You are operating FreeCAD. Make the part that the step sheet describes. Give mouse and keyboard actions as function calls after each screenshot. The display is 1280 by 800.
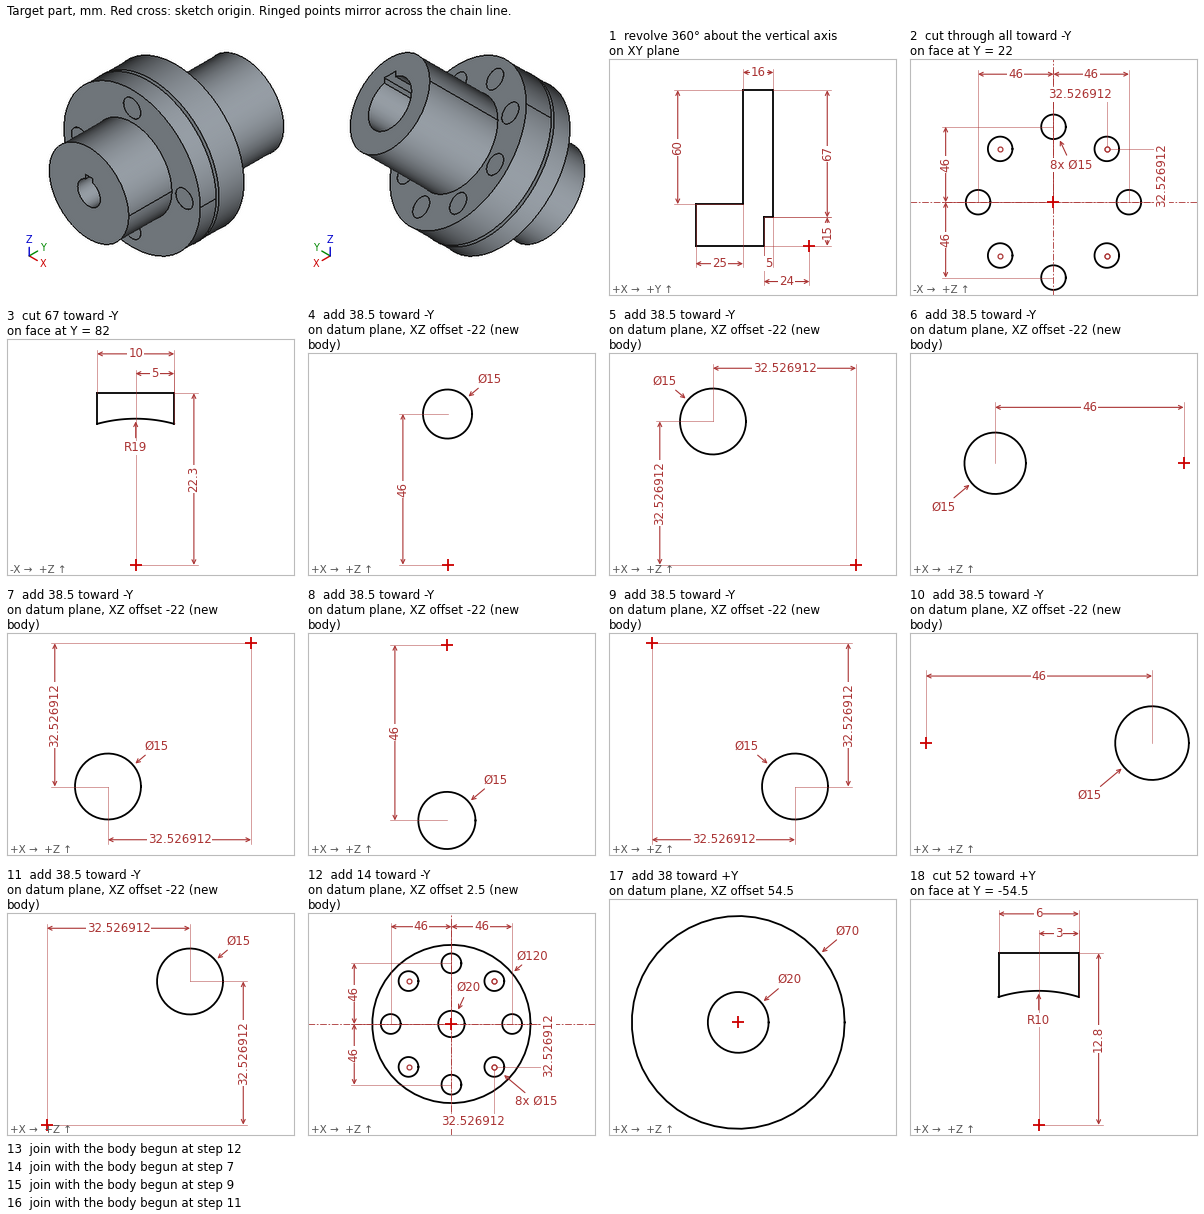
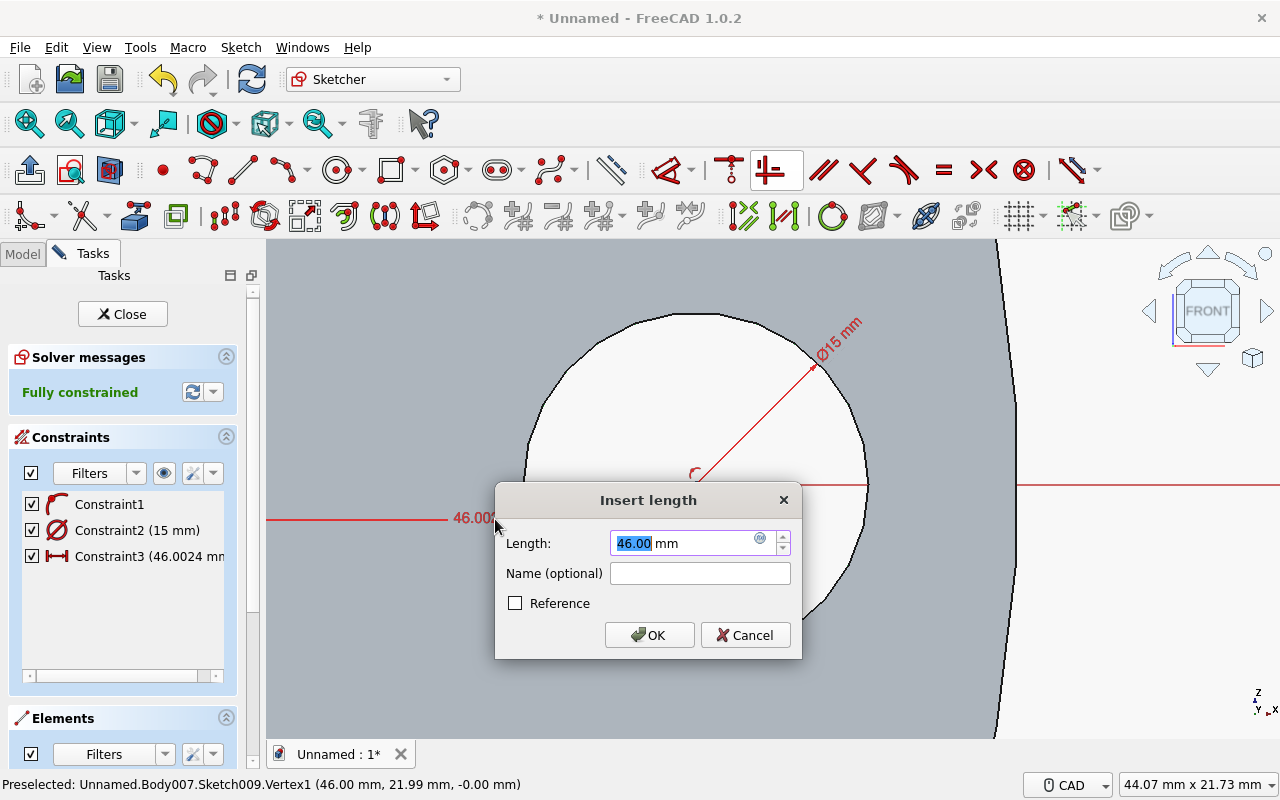
text(46)
key(Return)
key(Escape)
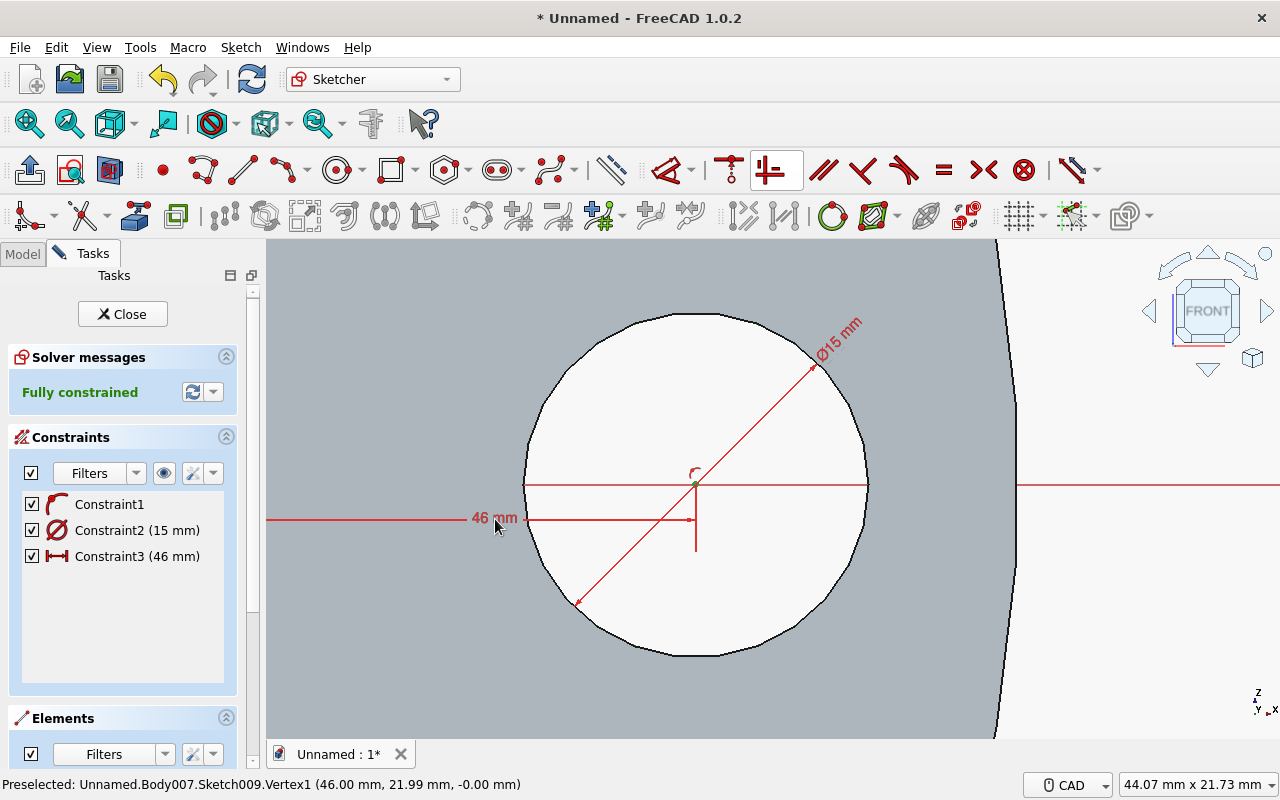
click(123, 314)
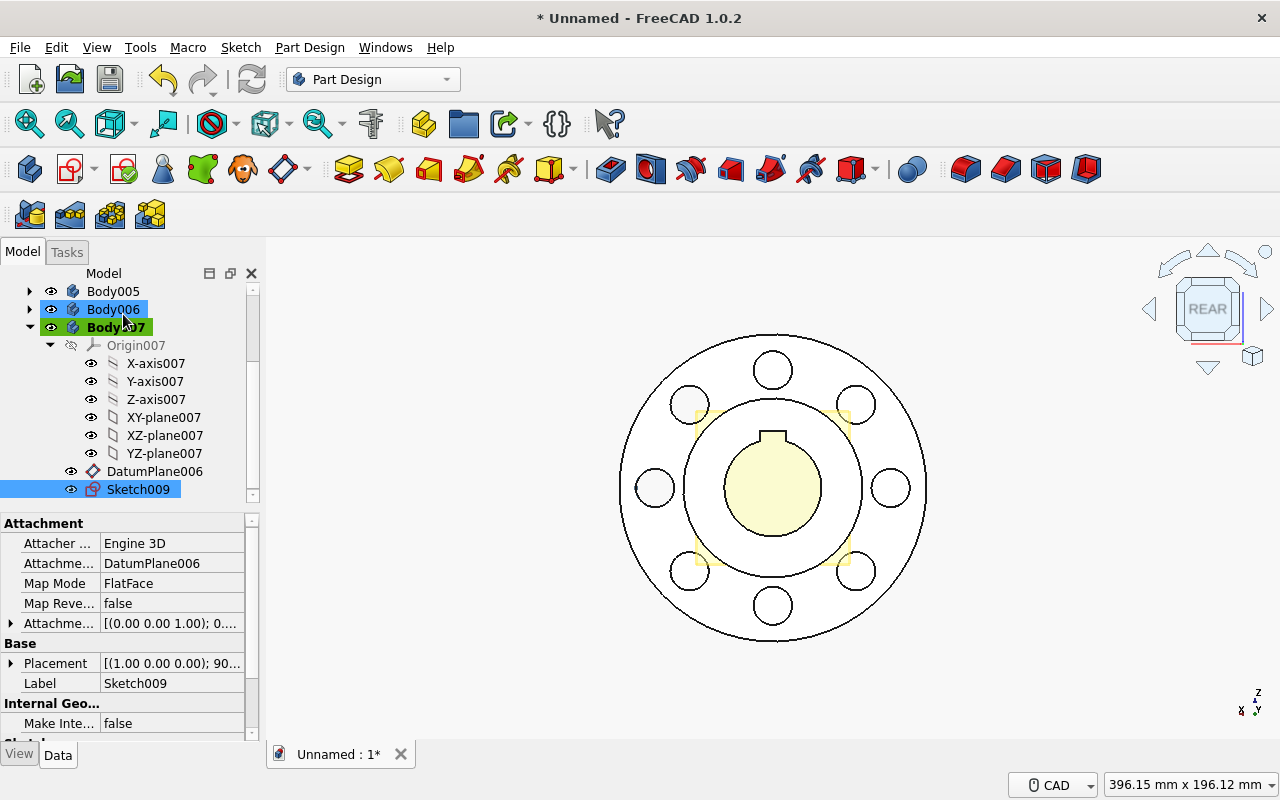
click(350, 170)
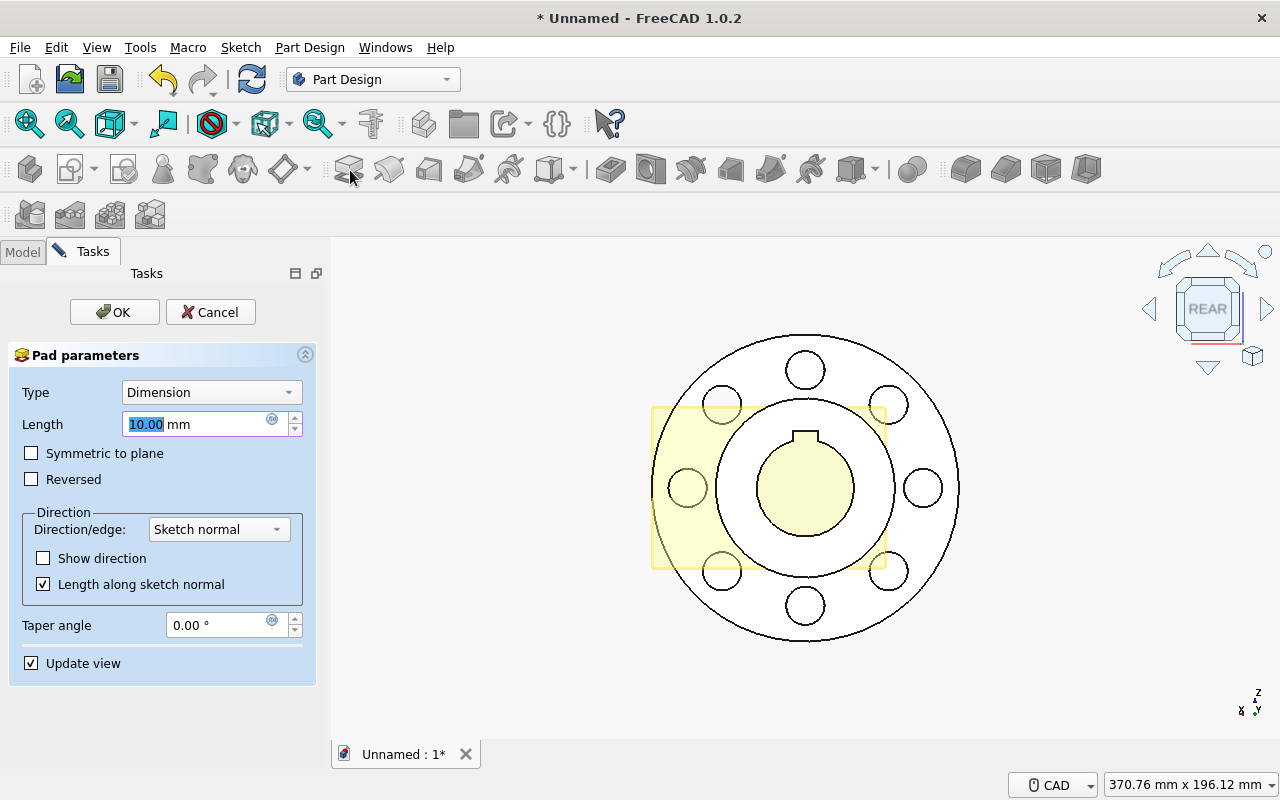
text(38.5)
key(Tab)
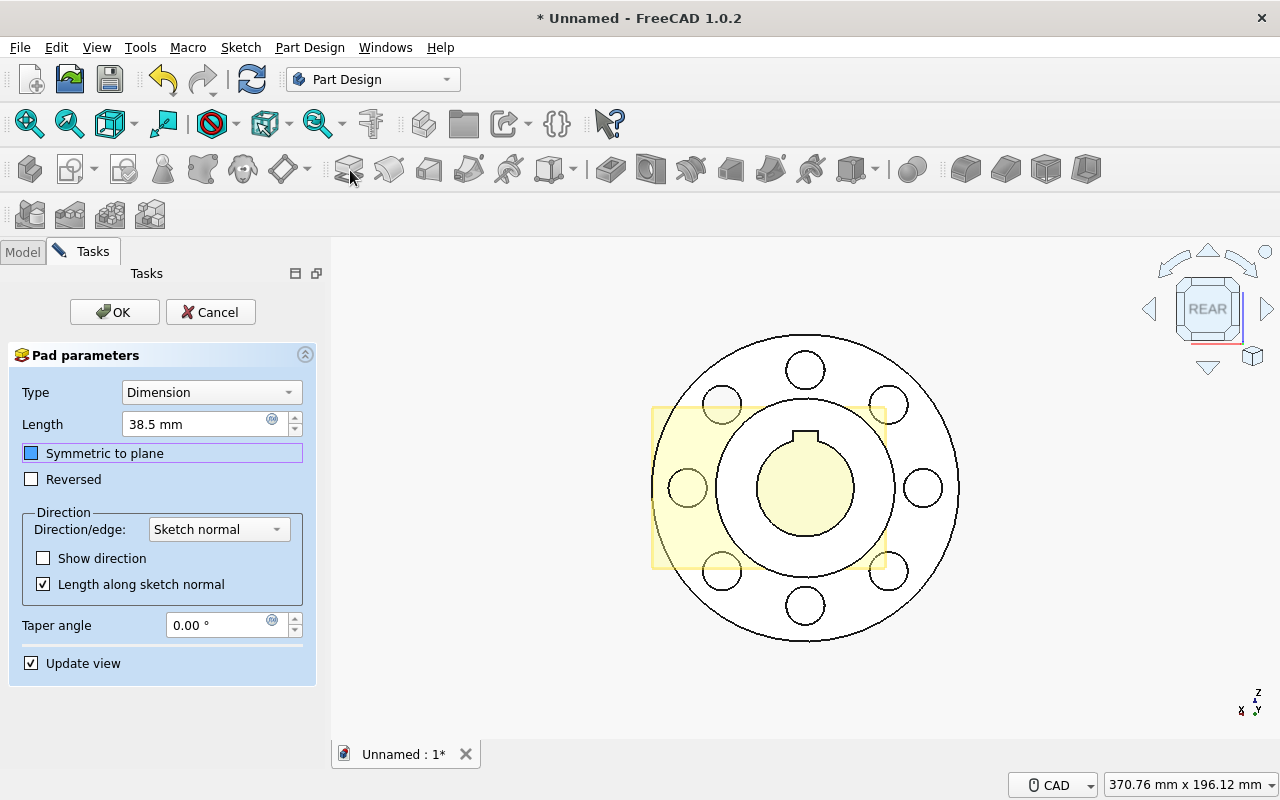
click(115, 312)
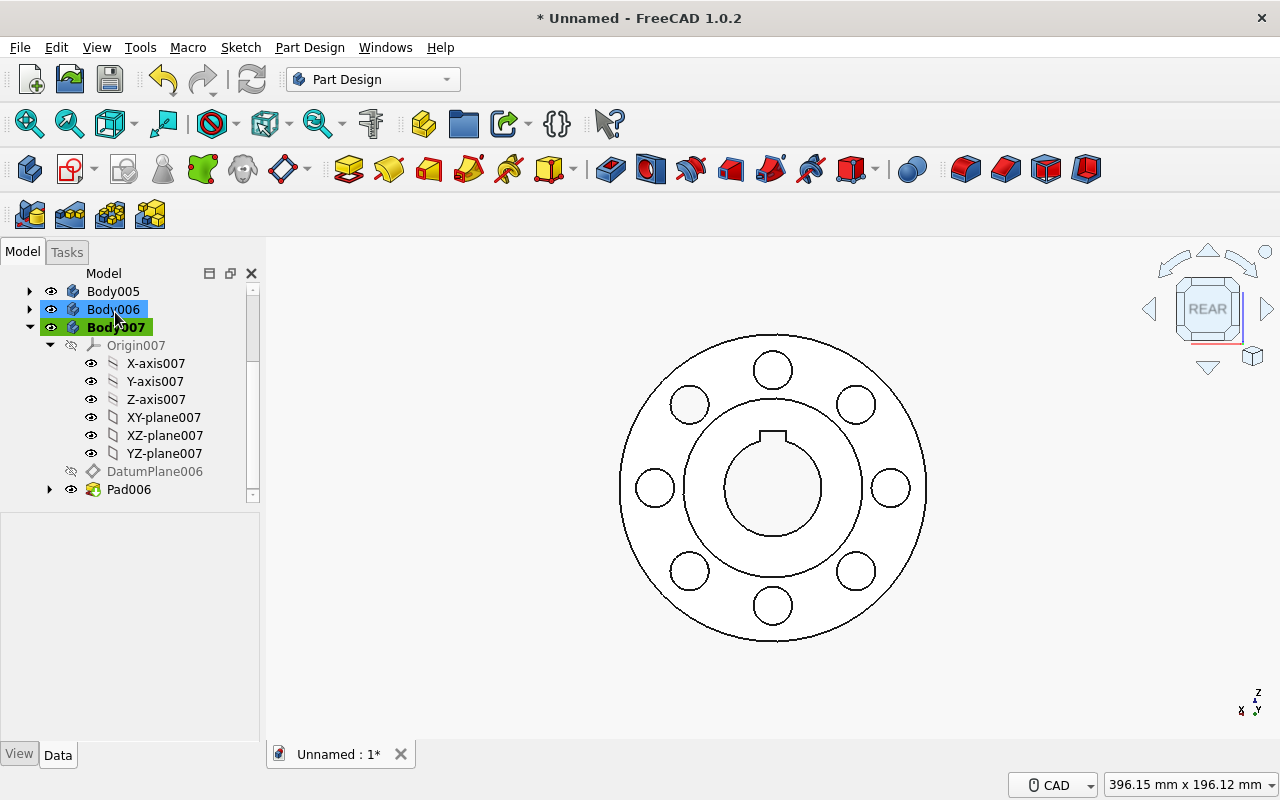
click(30, 124)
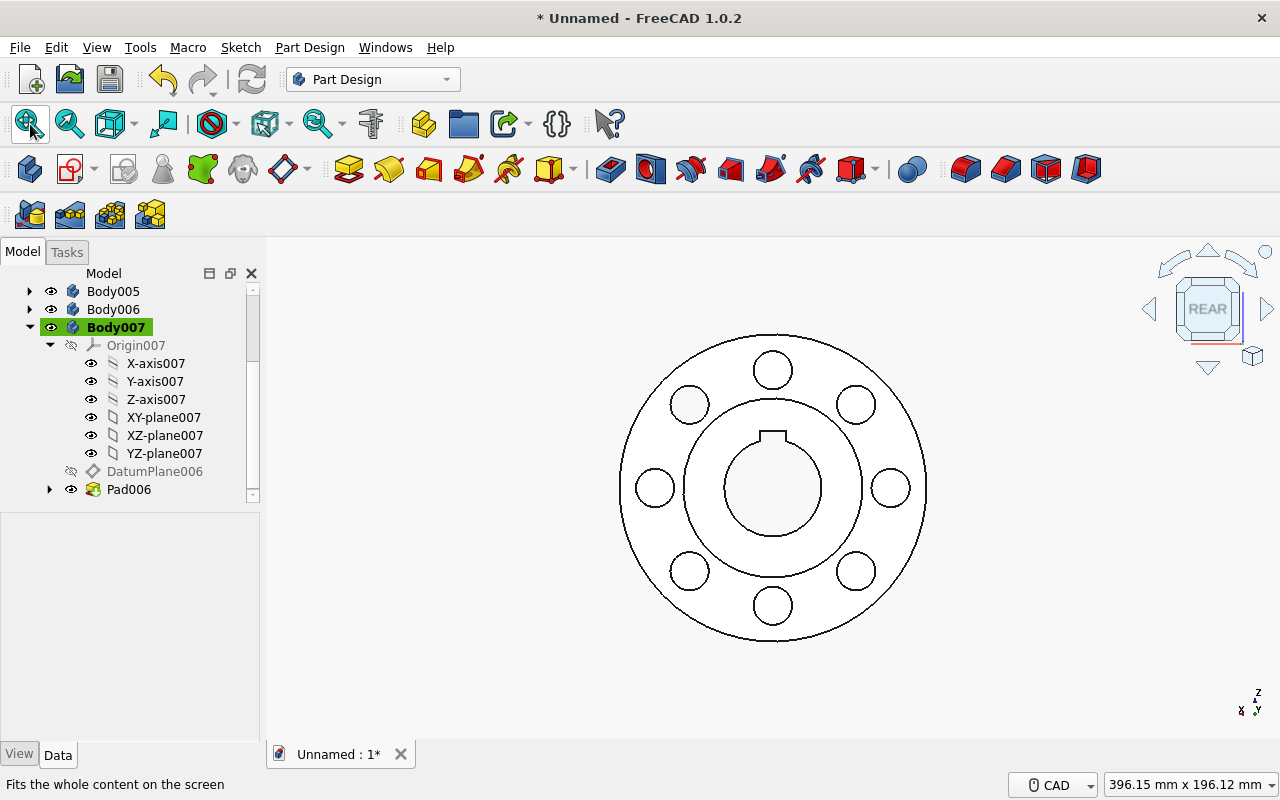
click(30, 170)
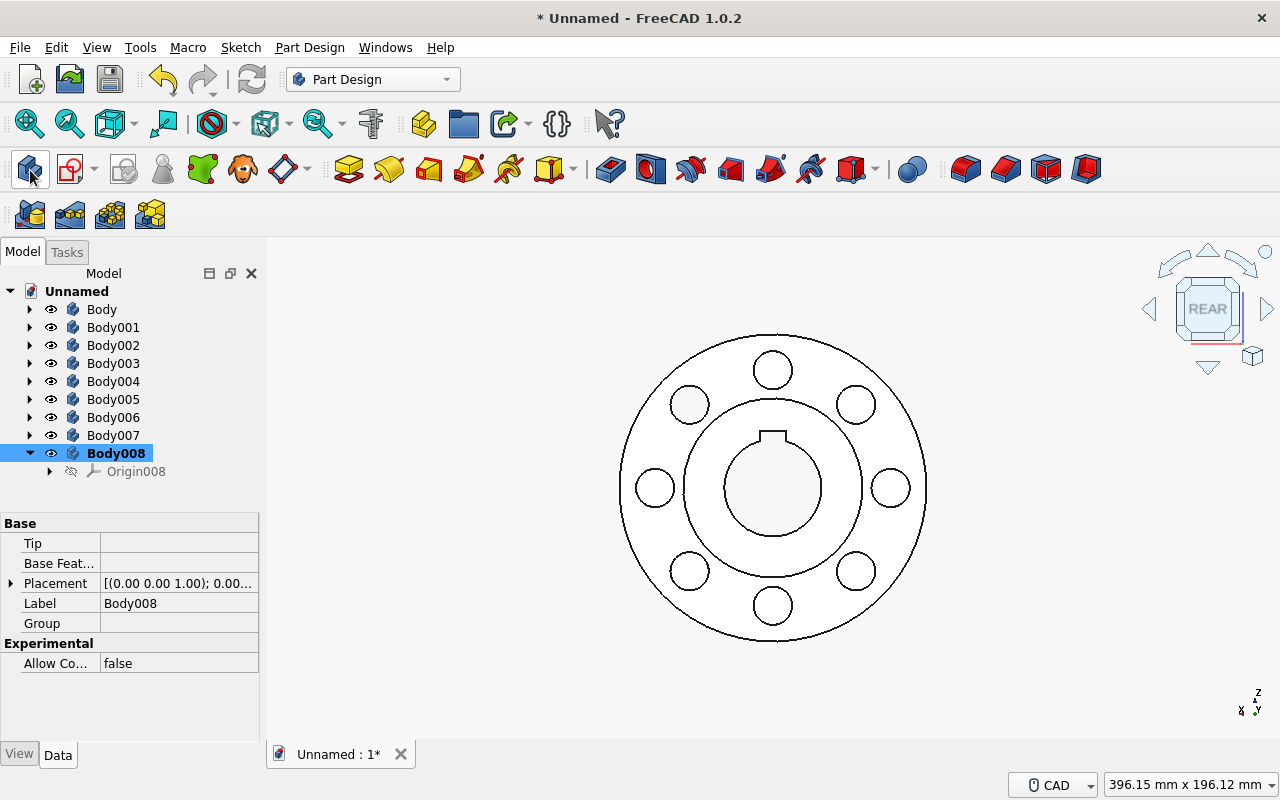
click(50, 471)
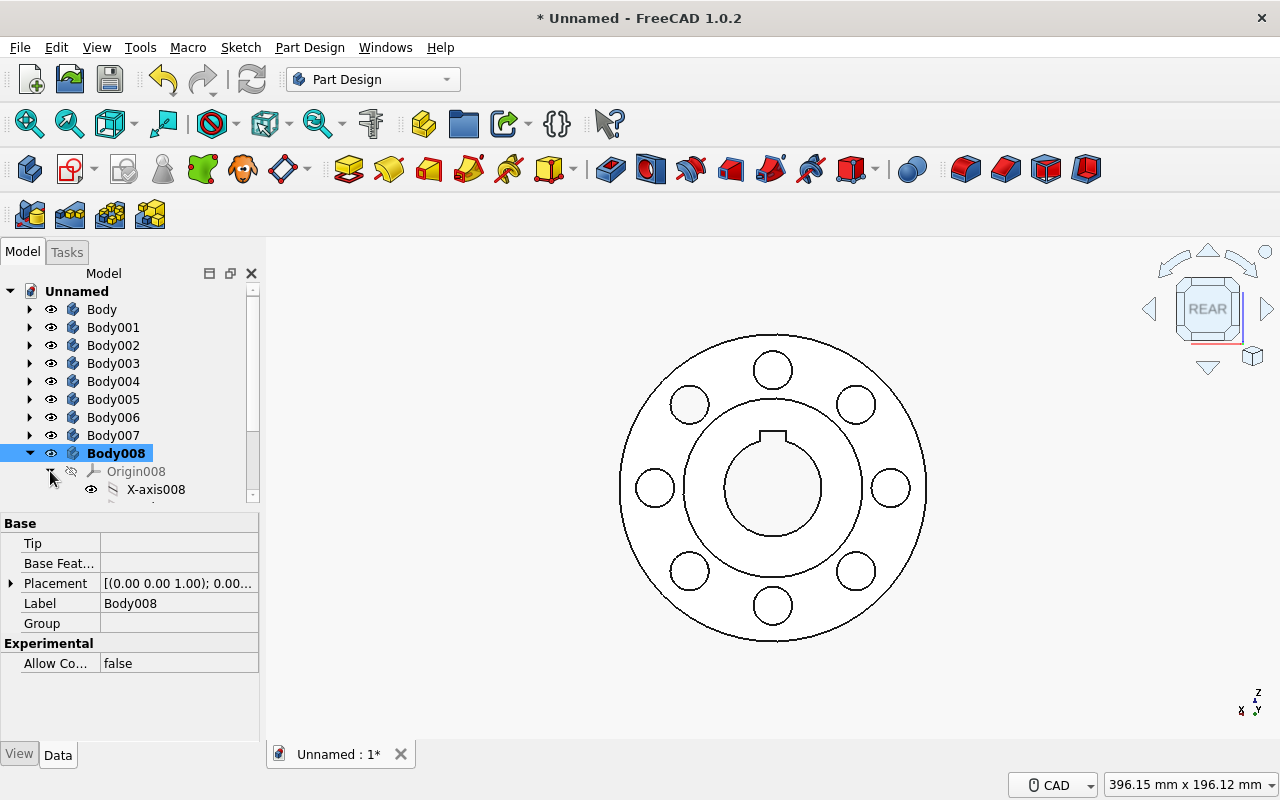
scroll(100, 395, down, 3)